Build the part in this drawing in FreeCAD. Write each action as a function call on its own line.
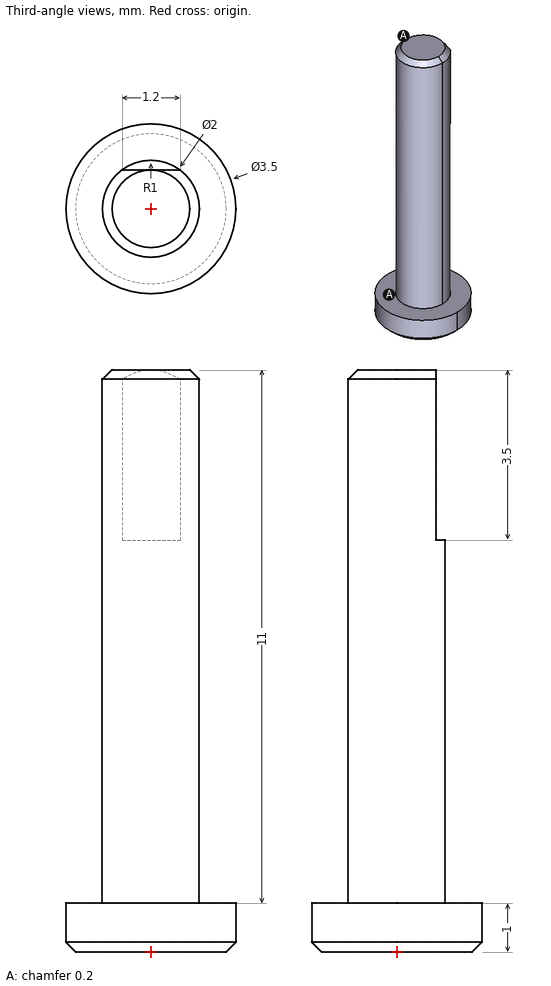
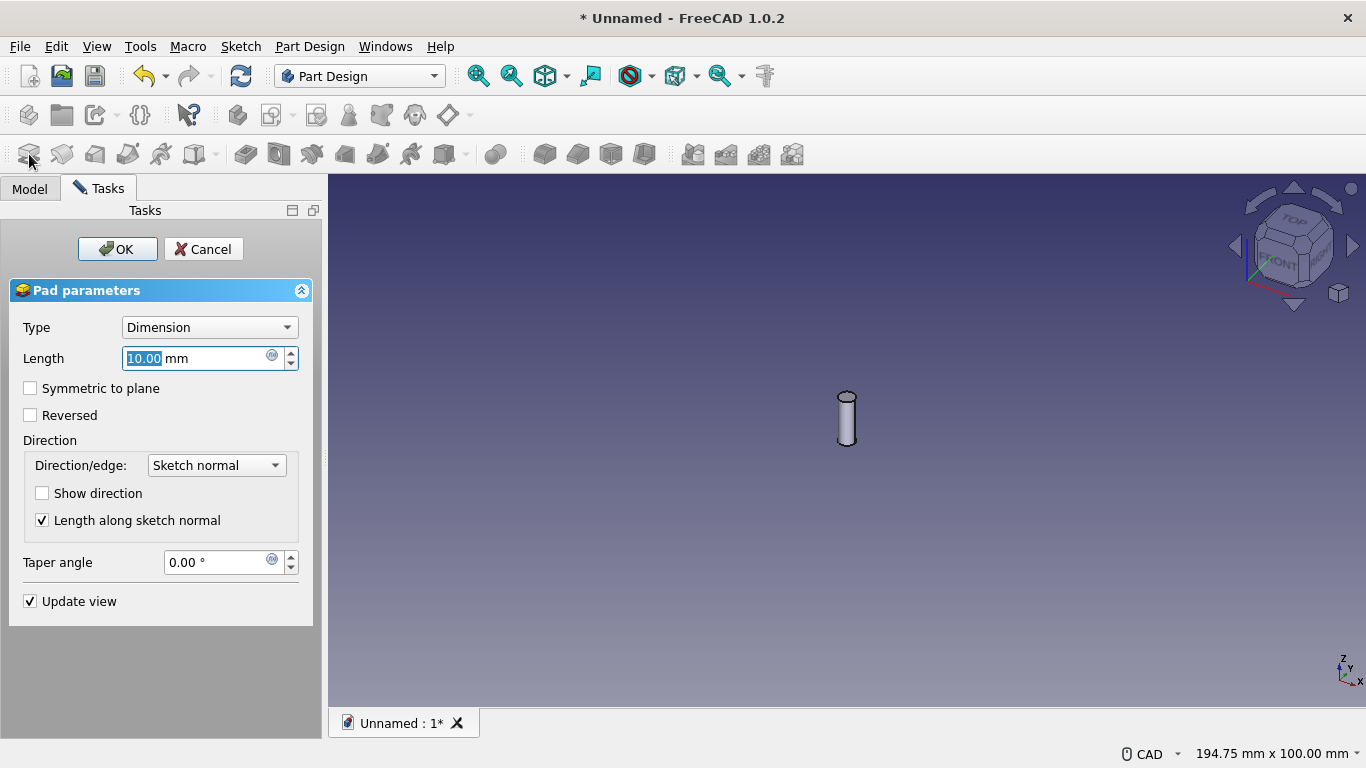
text(1)
key(Tab)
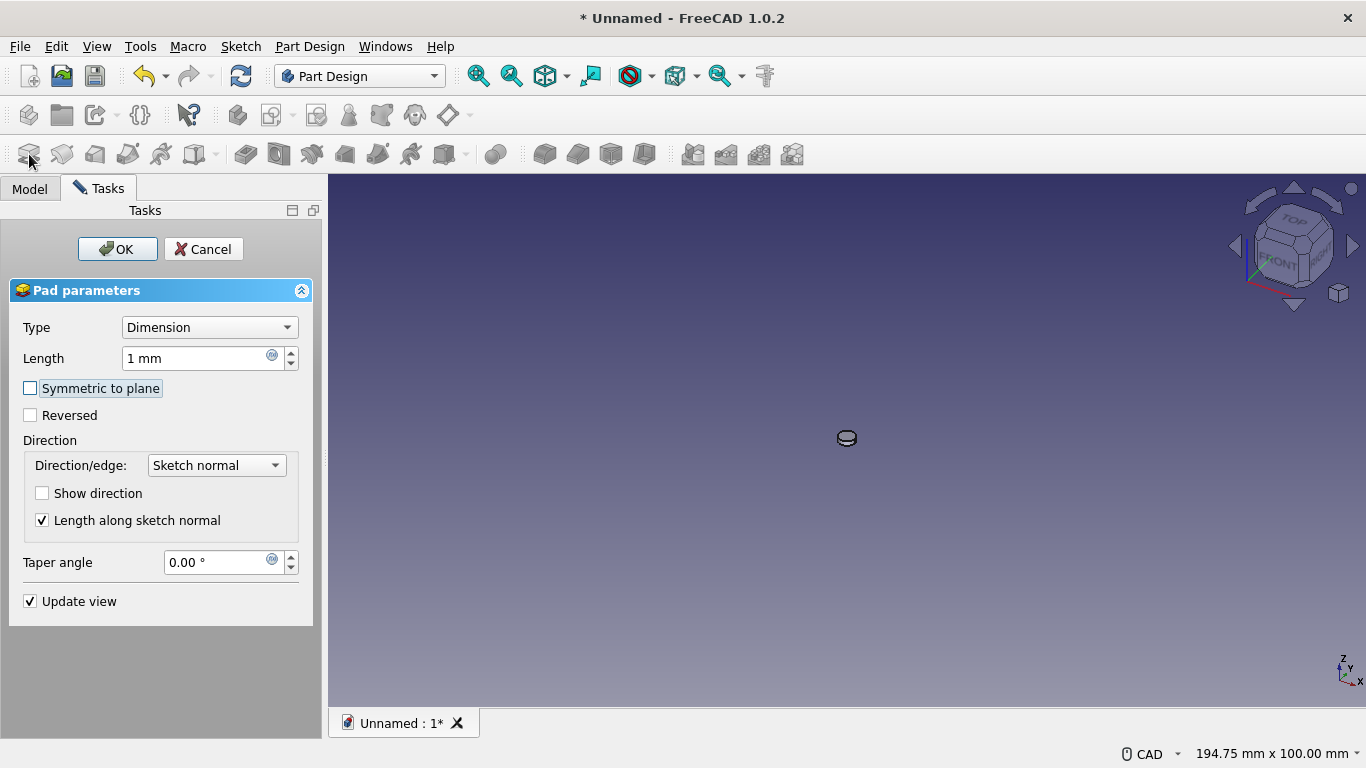
click(118, 249)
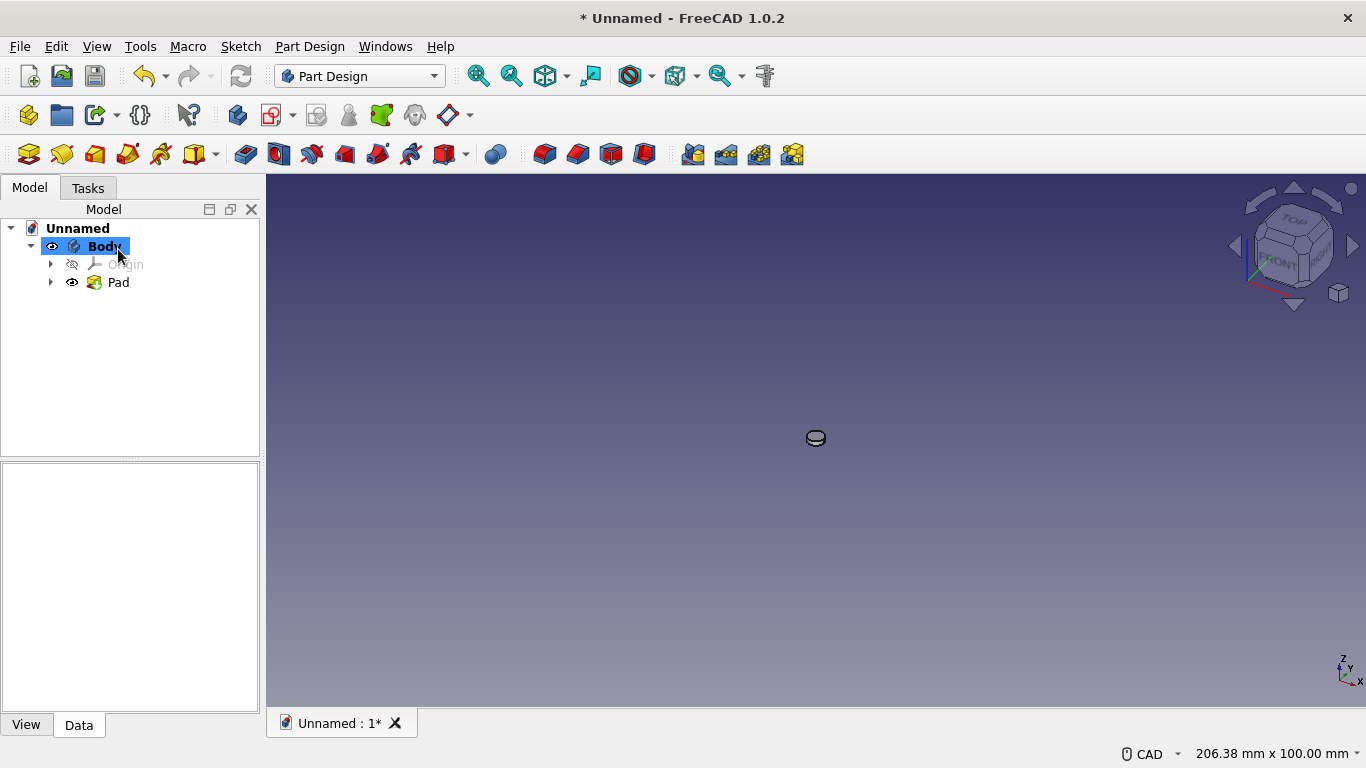
click(479, 76)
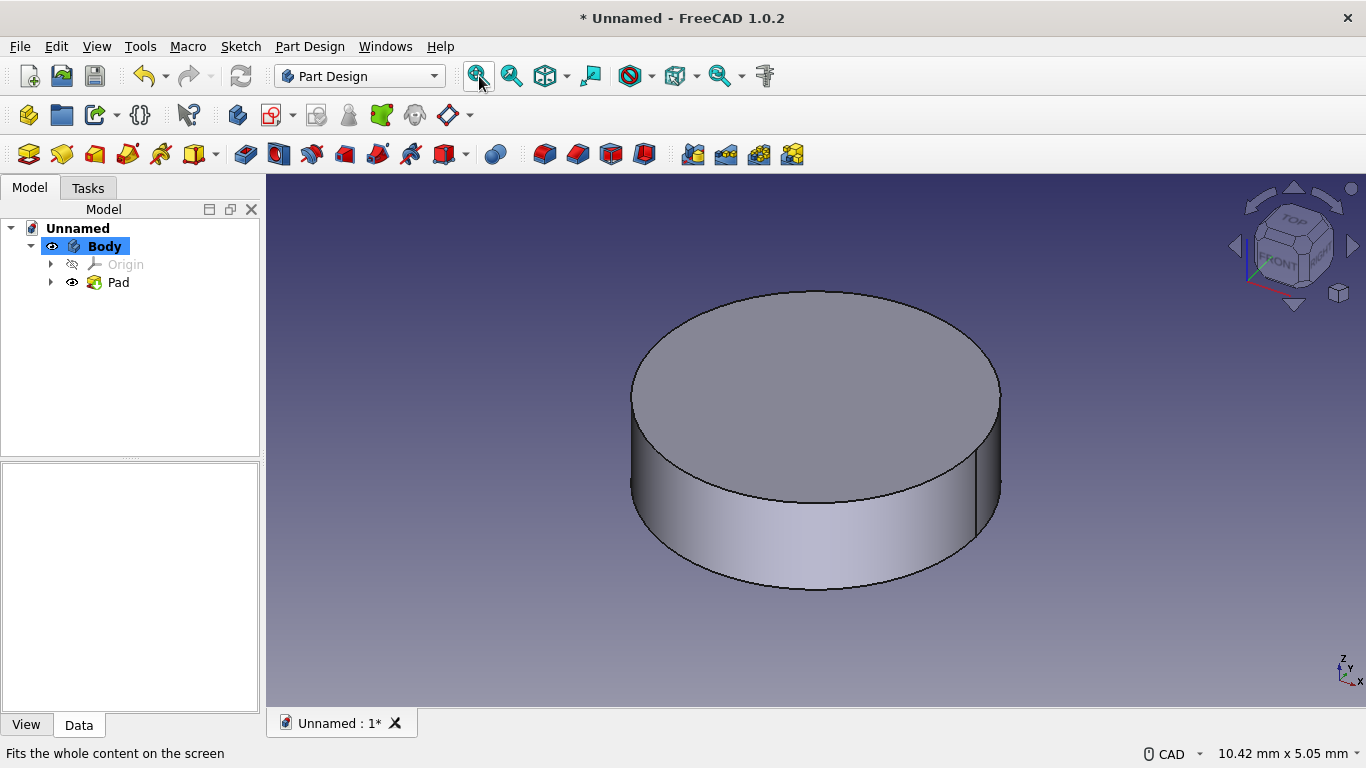
click(816, 396)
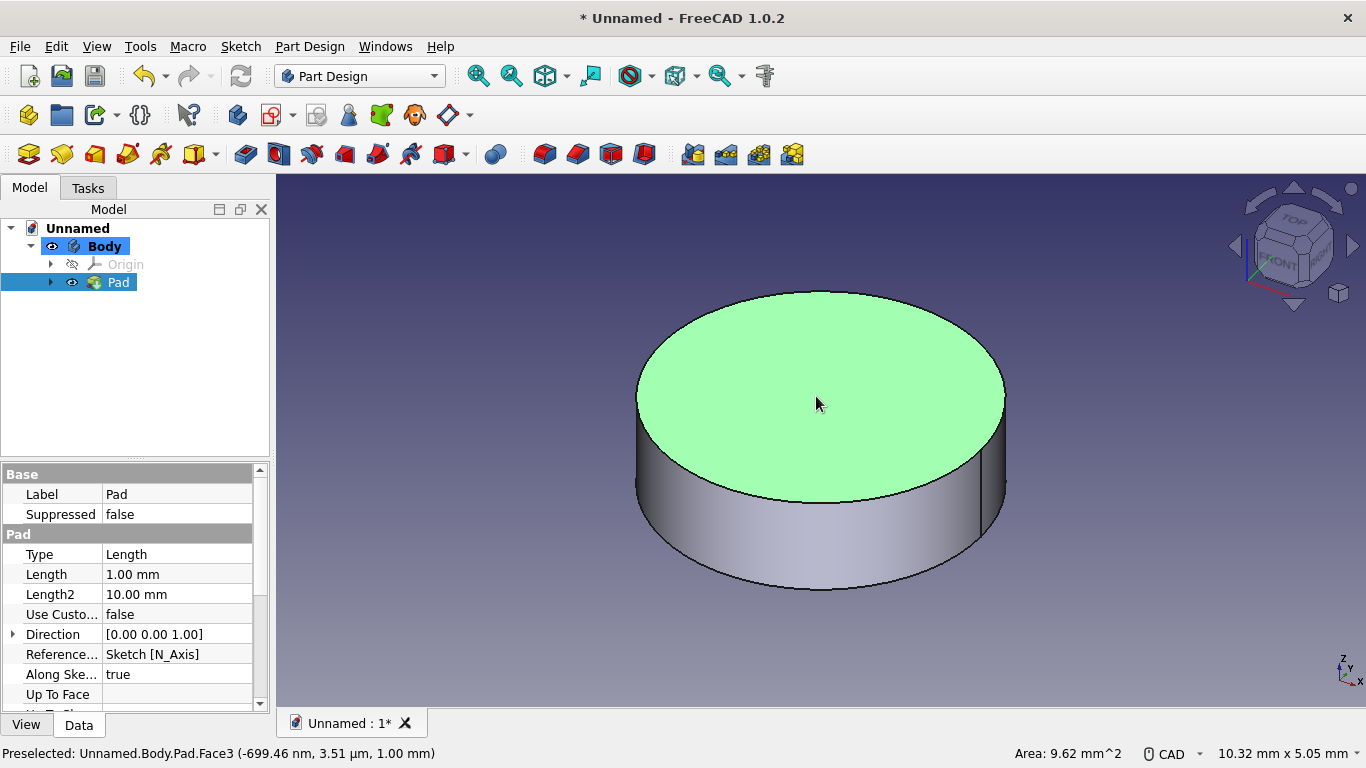
click(270, 116)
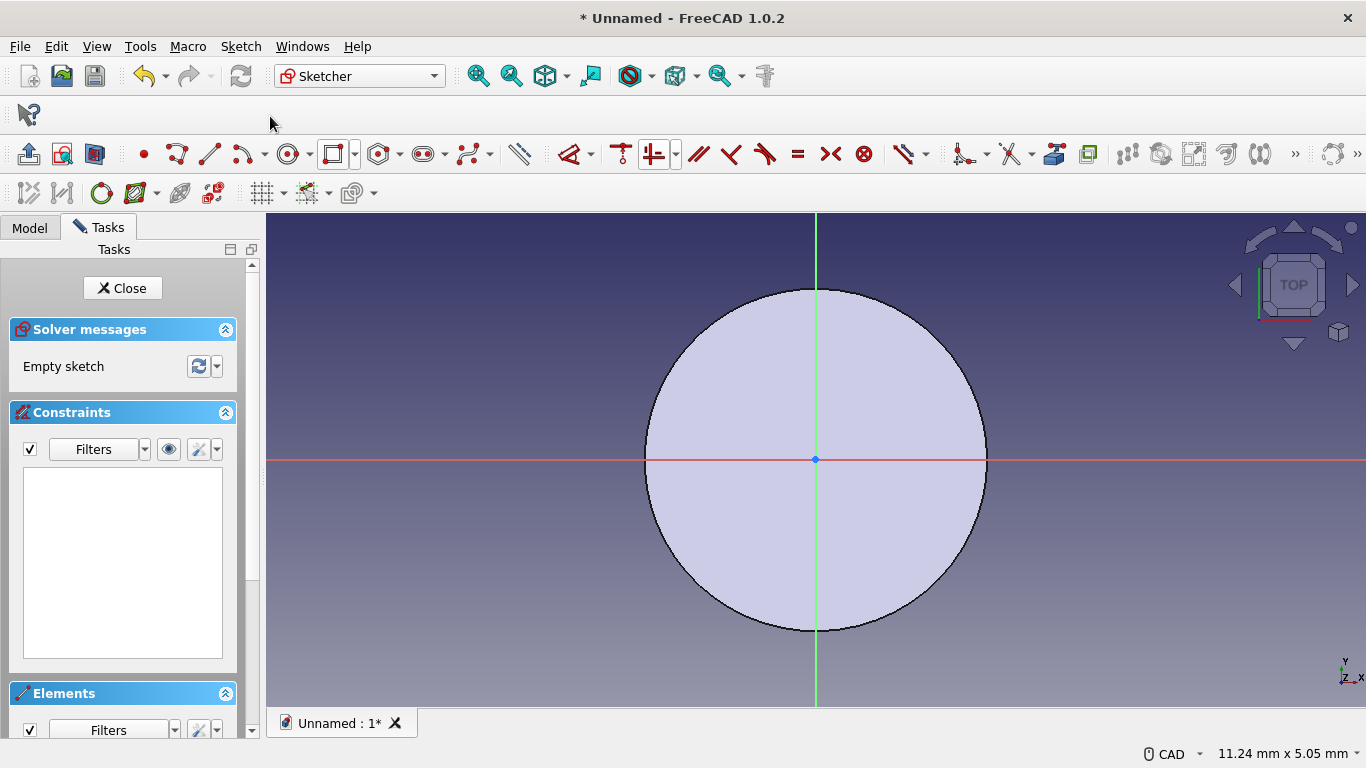
scroll(955, 460, up, 2)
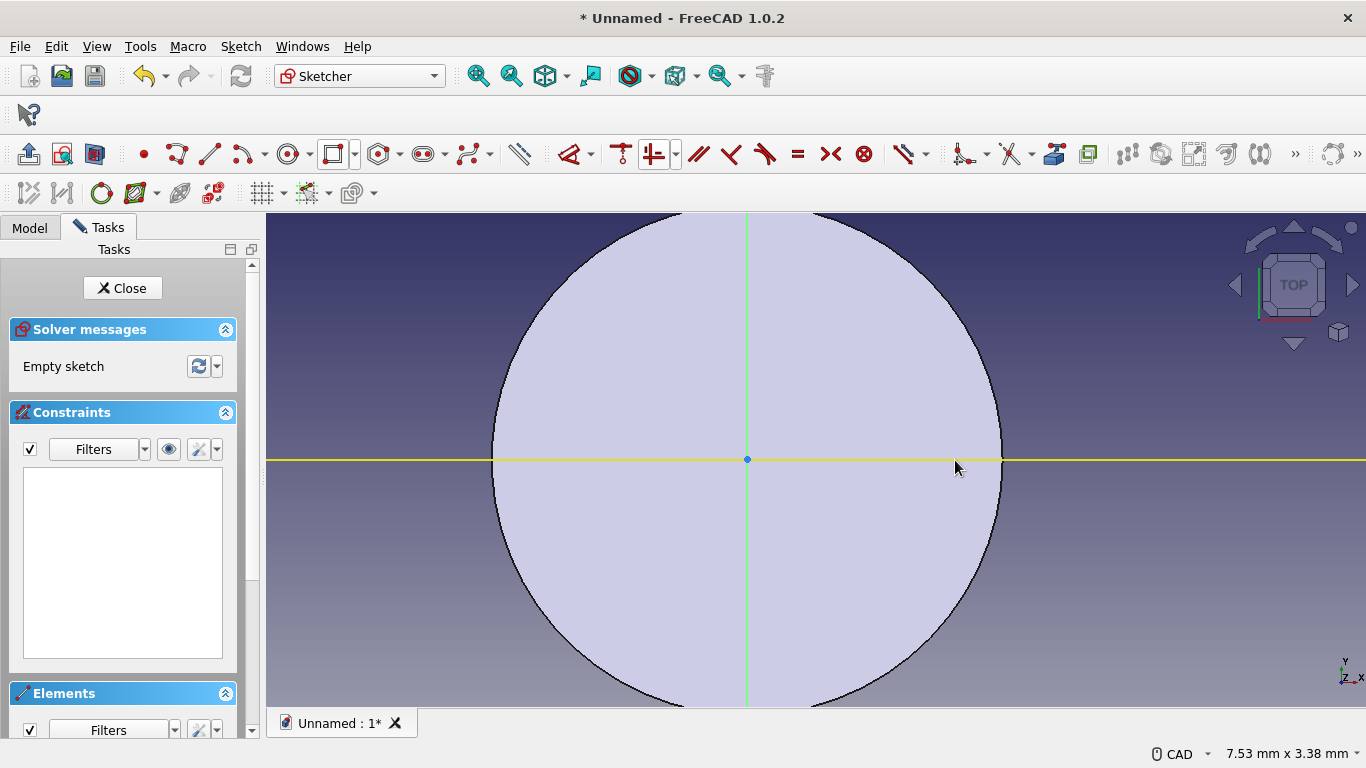
click(288, 154)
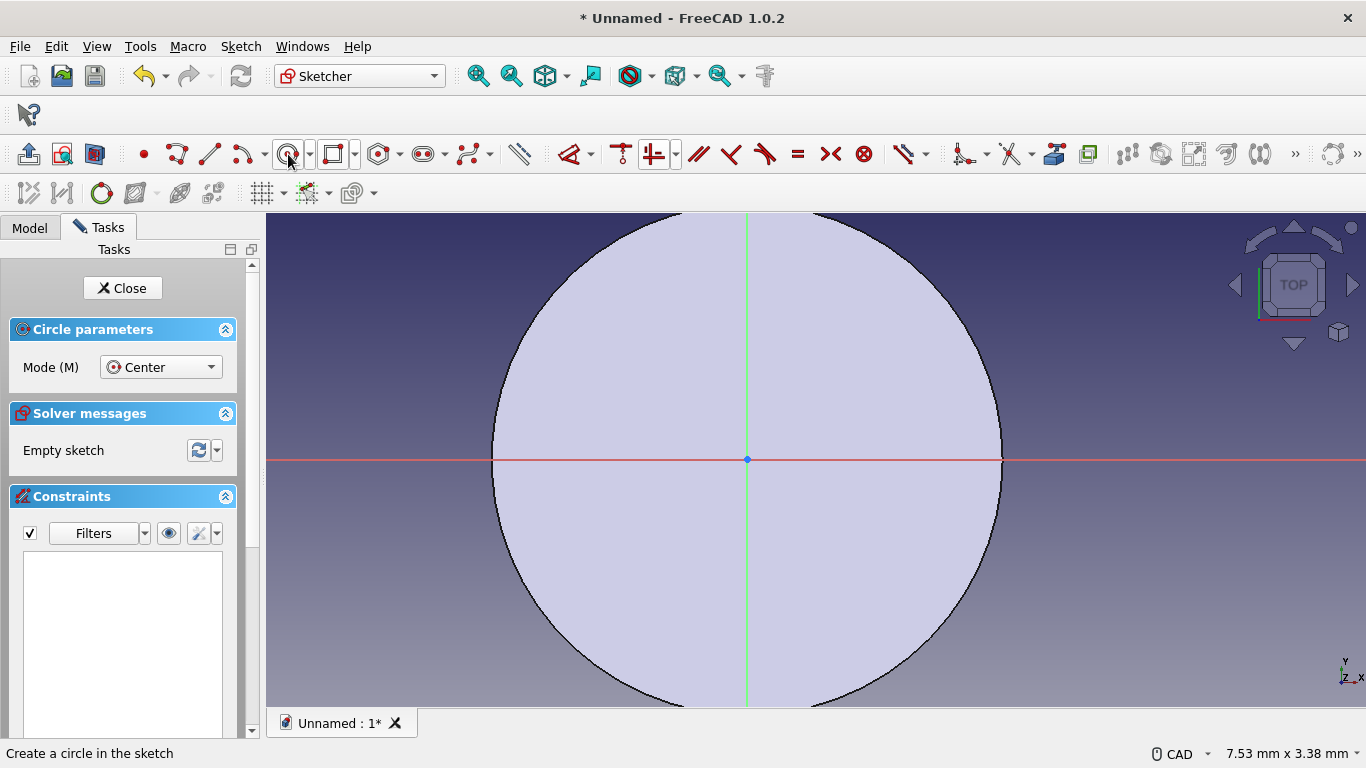
click(747, 460)
move(850, 357)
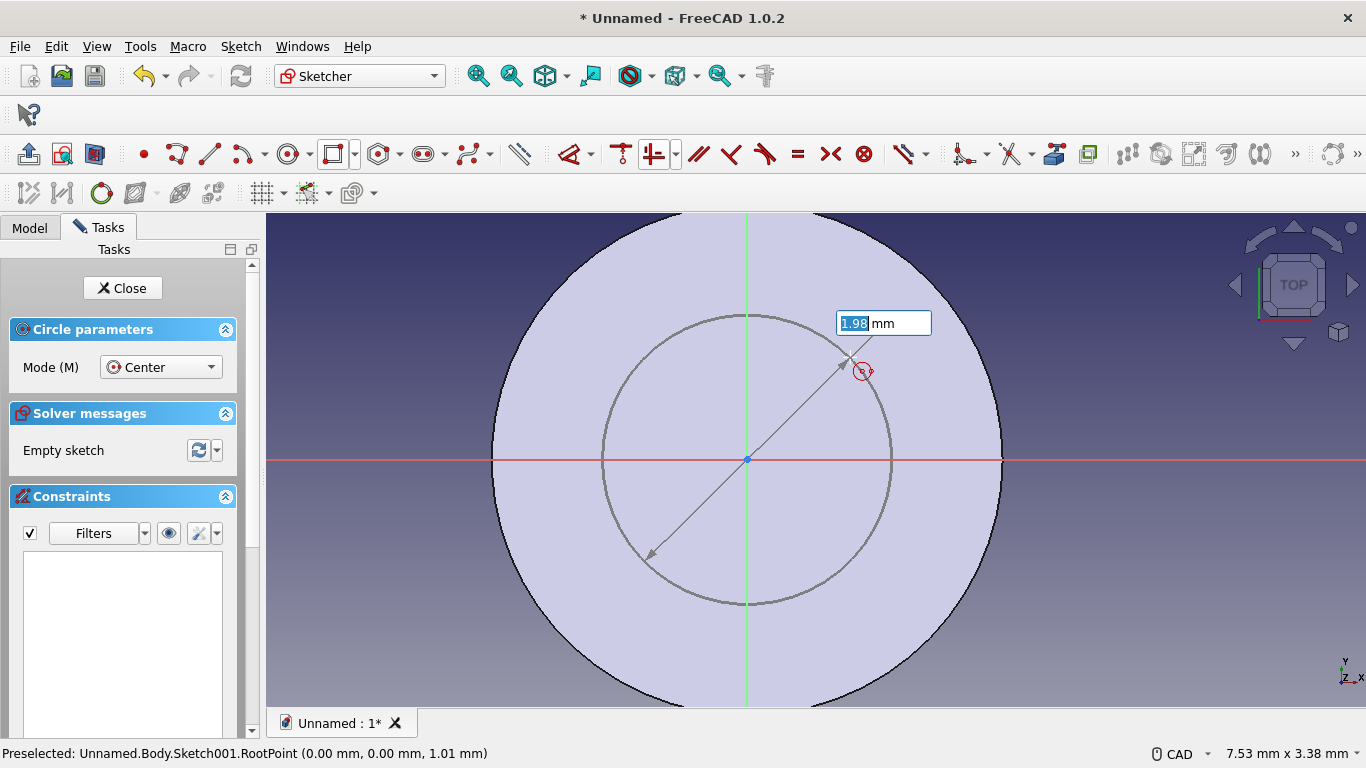
text(2)
key(Return)
key(Escape)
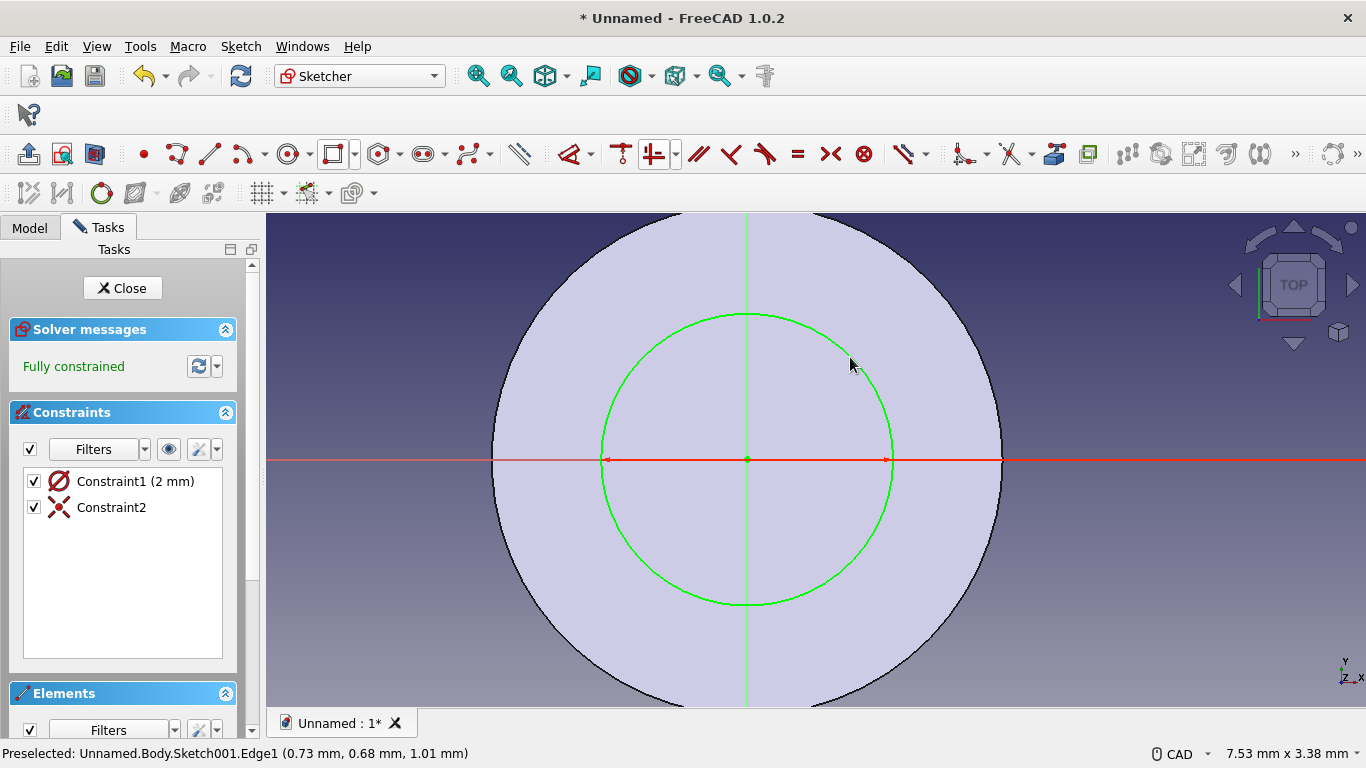
click(123, 288)